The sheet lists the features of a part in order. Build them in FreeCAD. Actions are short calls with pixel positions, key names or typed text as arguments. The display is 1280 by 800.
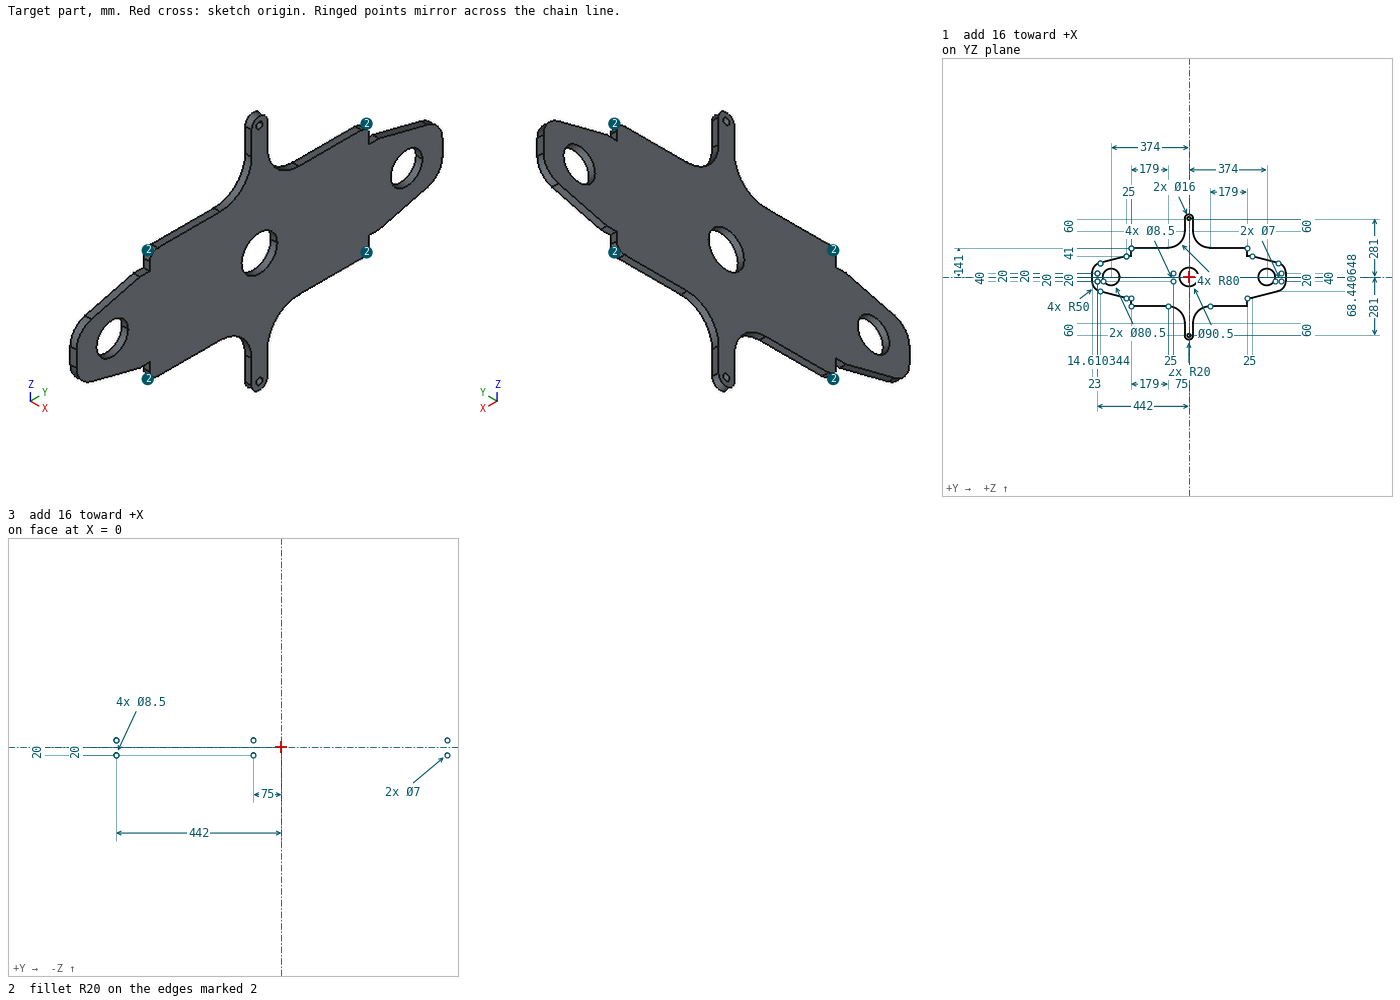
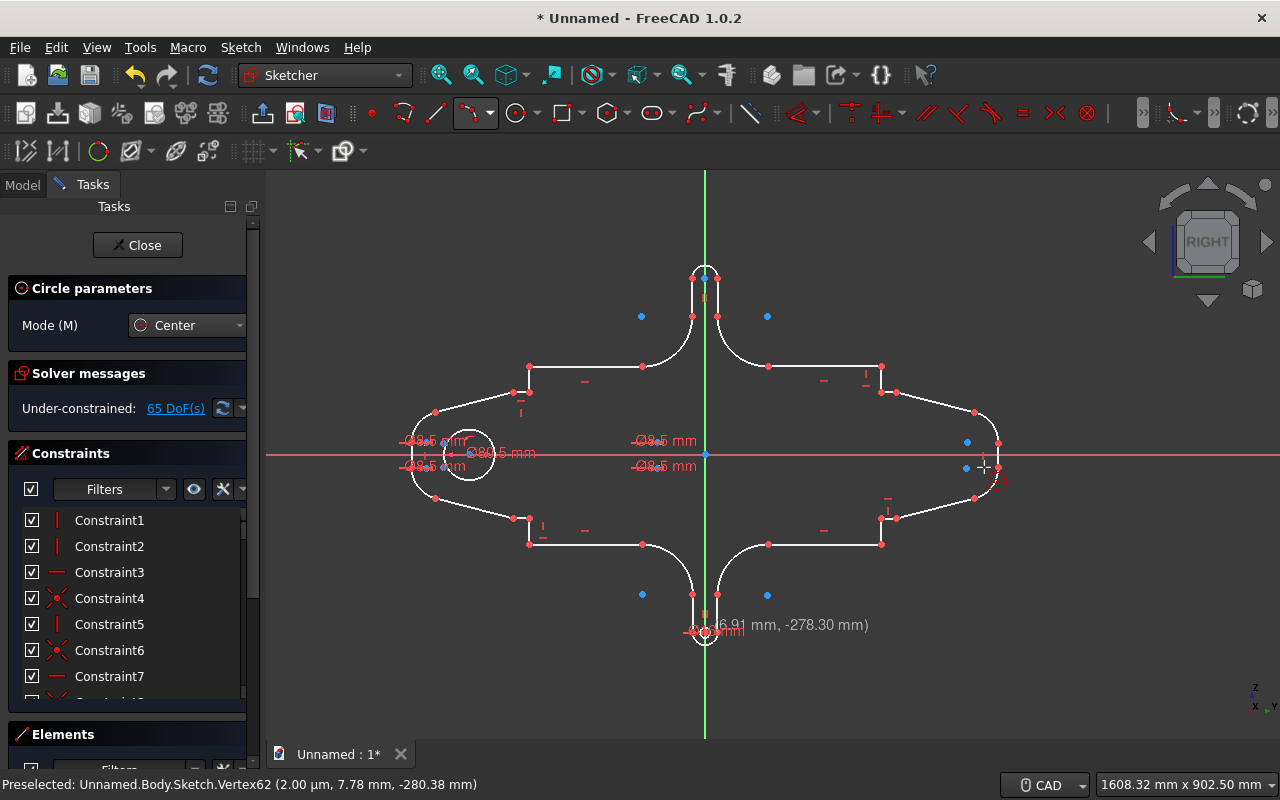
scroll(984, 467, up, 2)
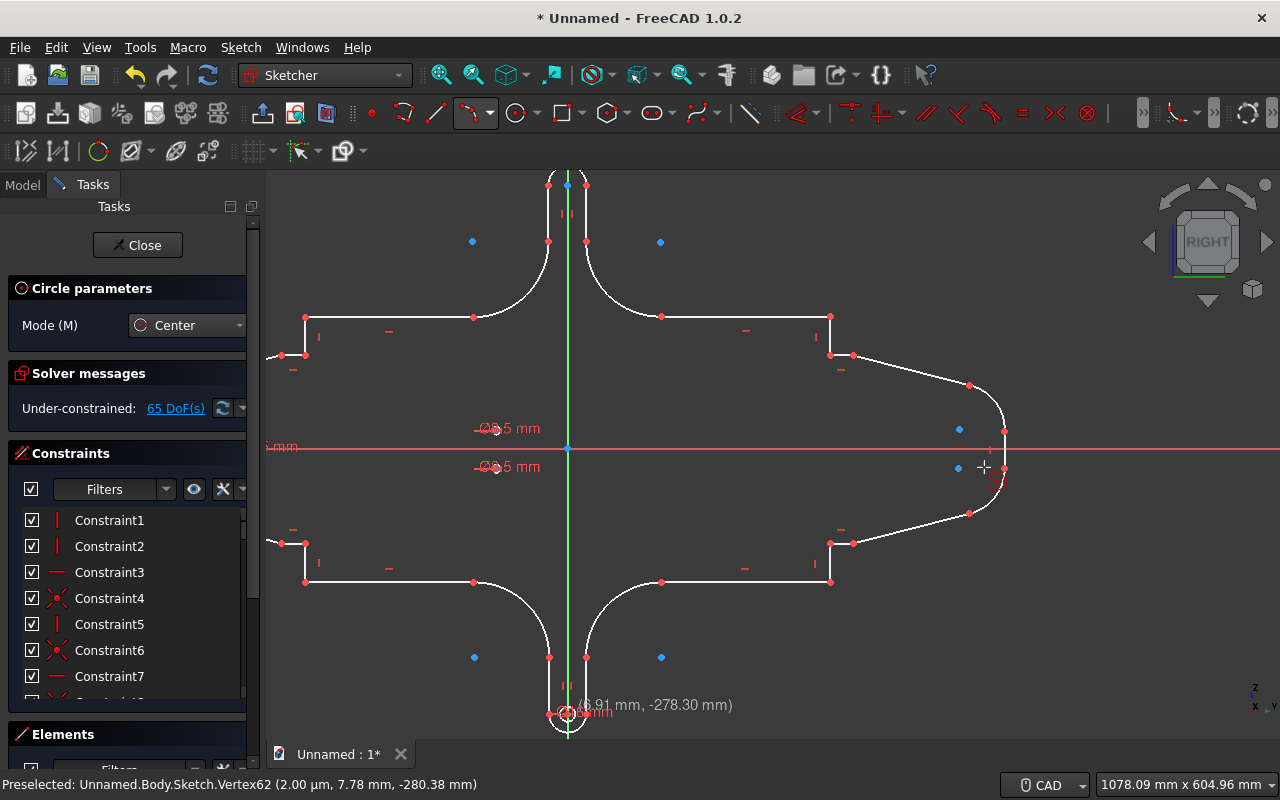
click(983, 467)
move(986, 465)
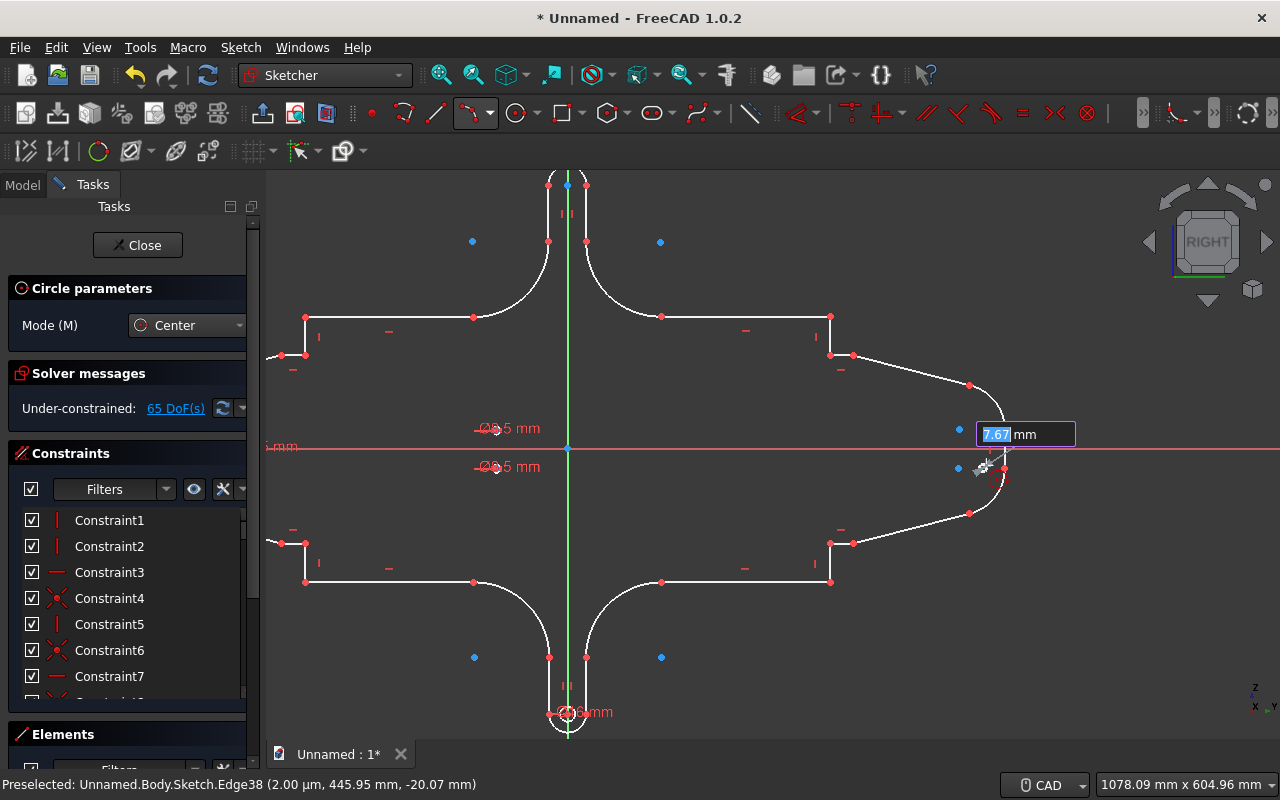
text(7)
key(Return)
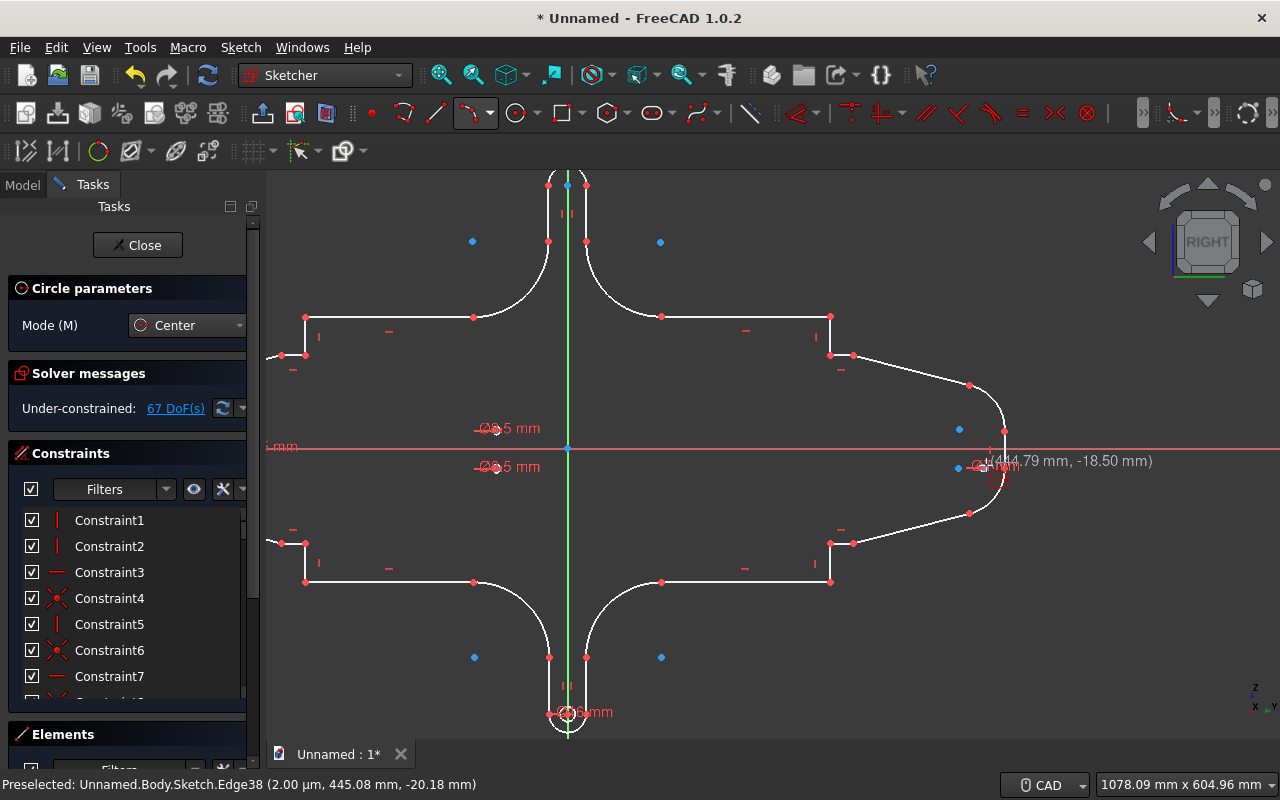
click(568, 449)
move(598, 419)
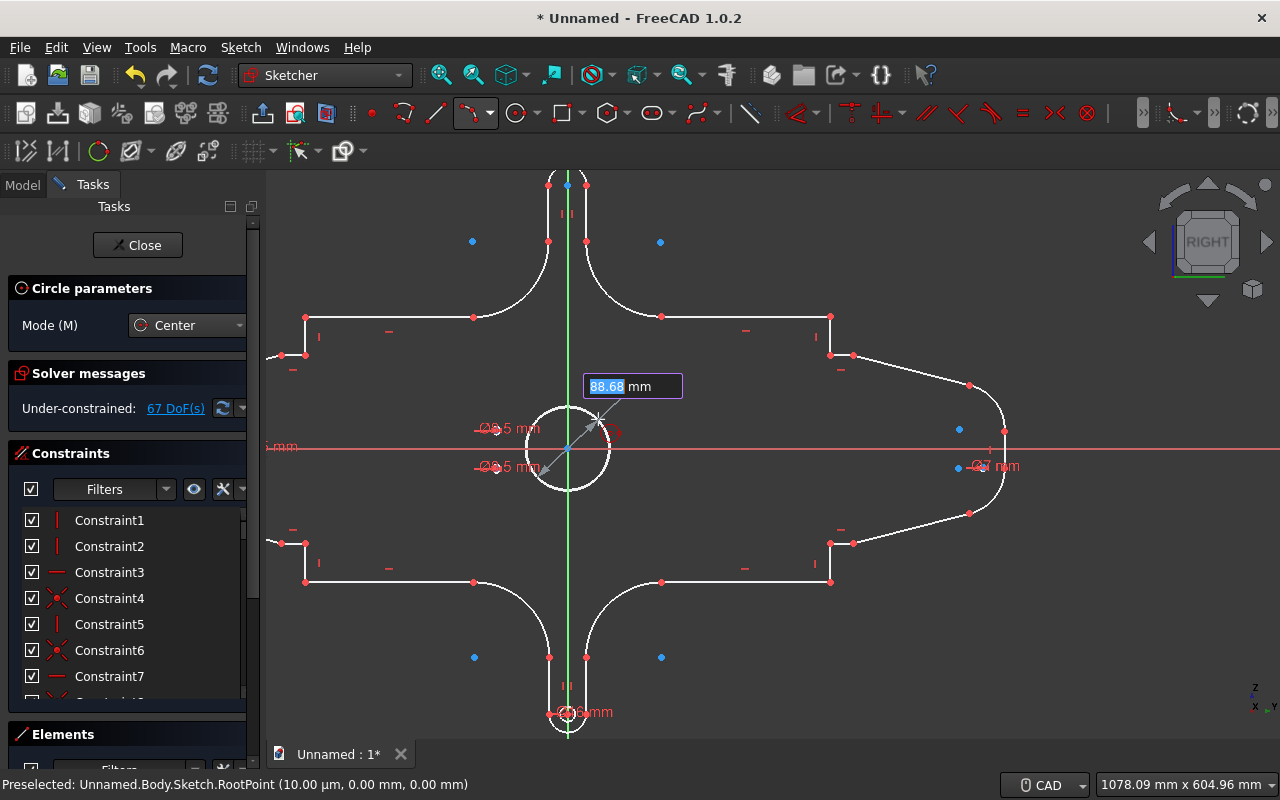
text(90.5)
key(Return)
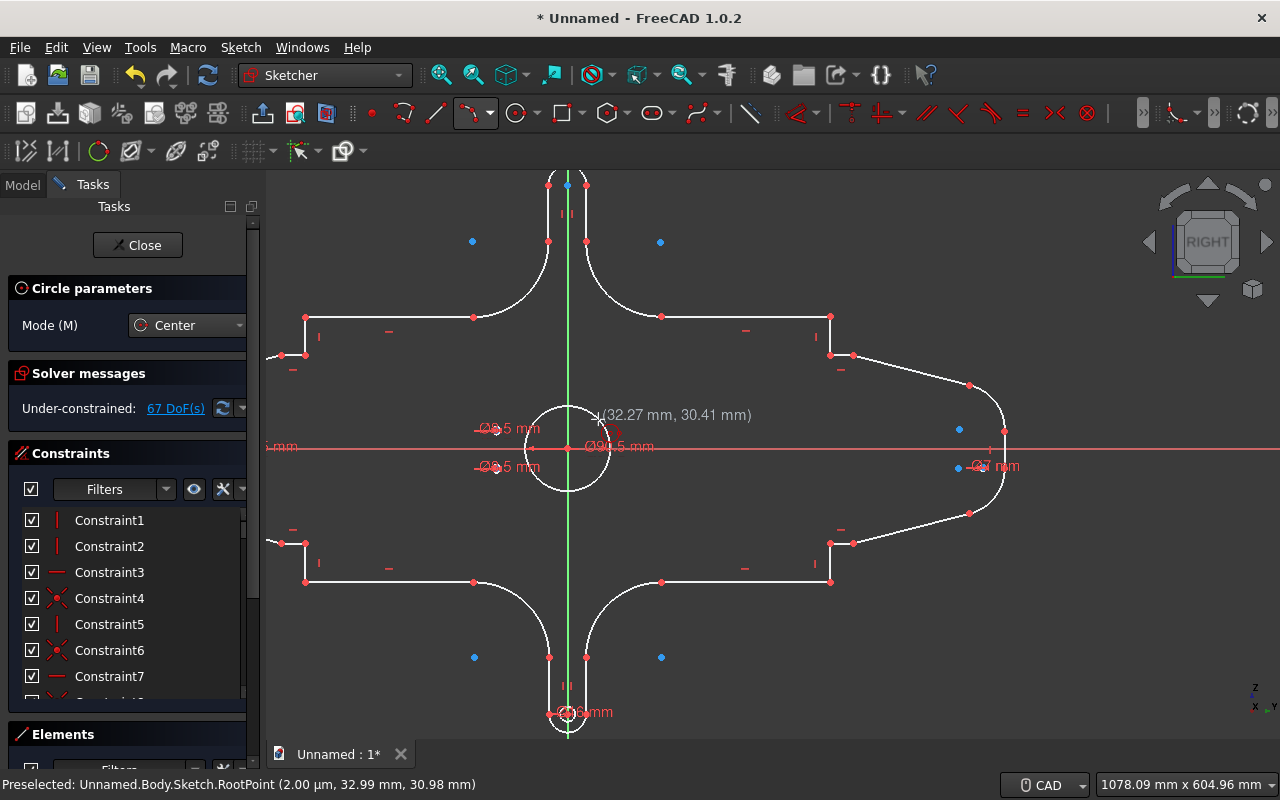
scroll(983, 466, down, 2)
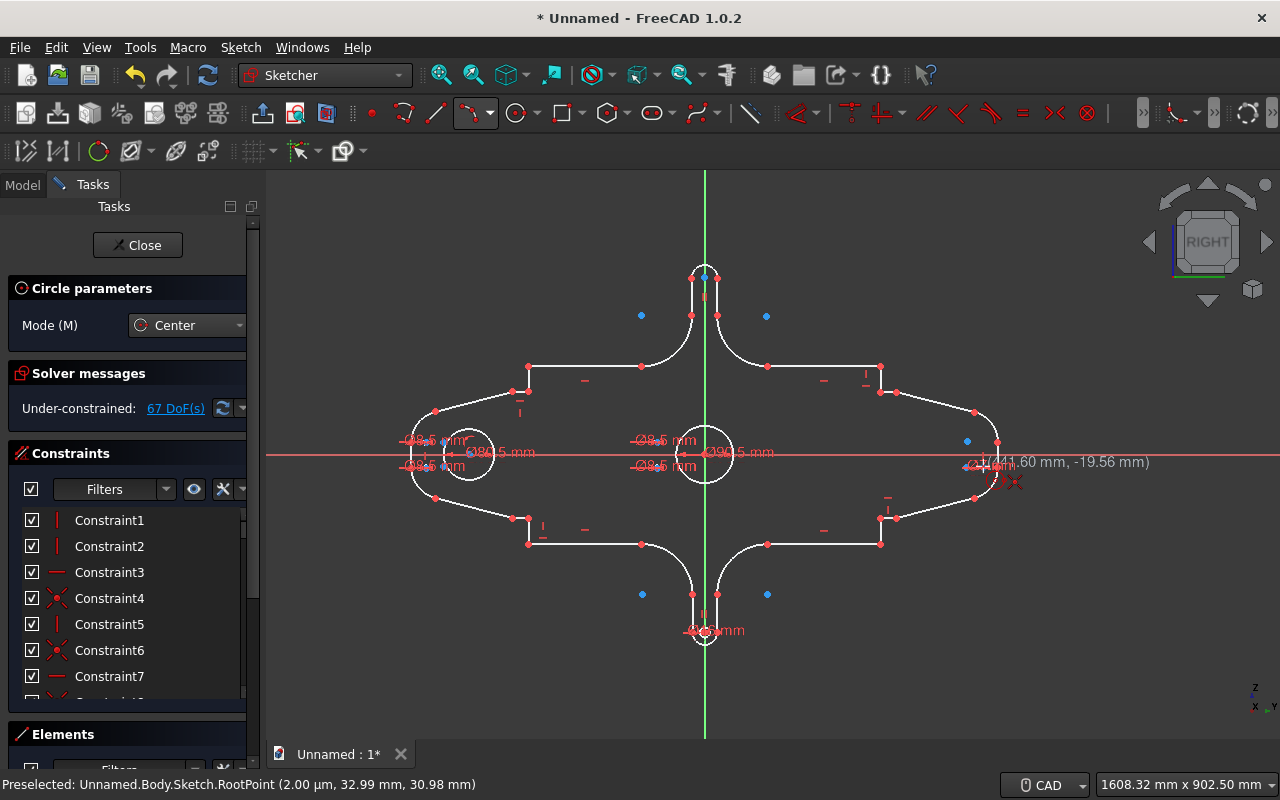
scroll(705, 277, up, 8)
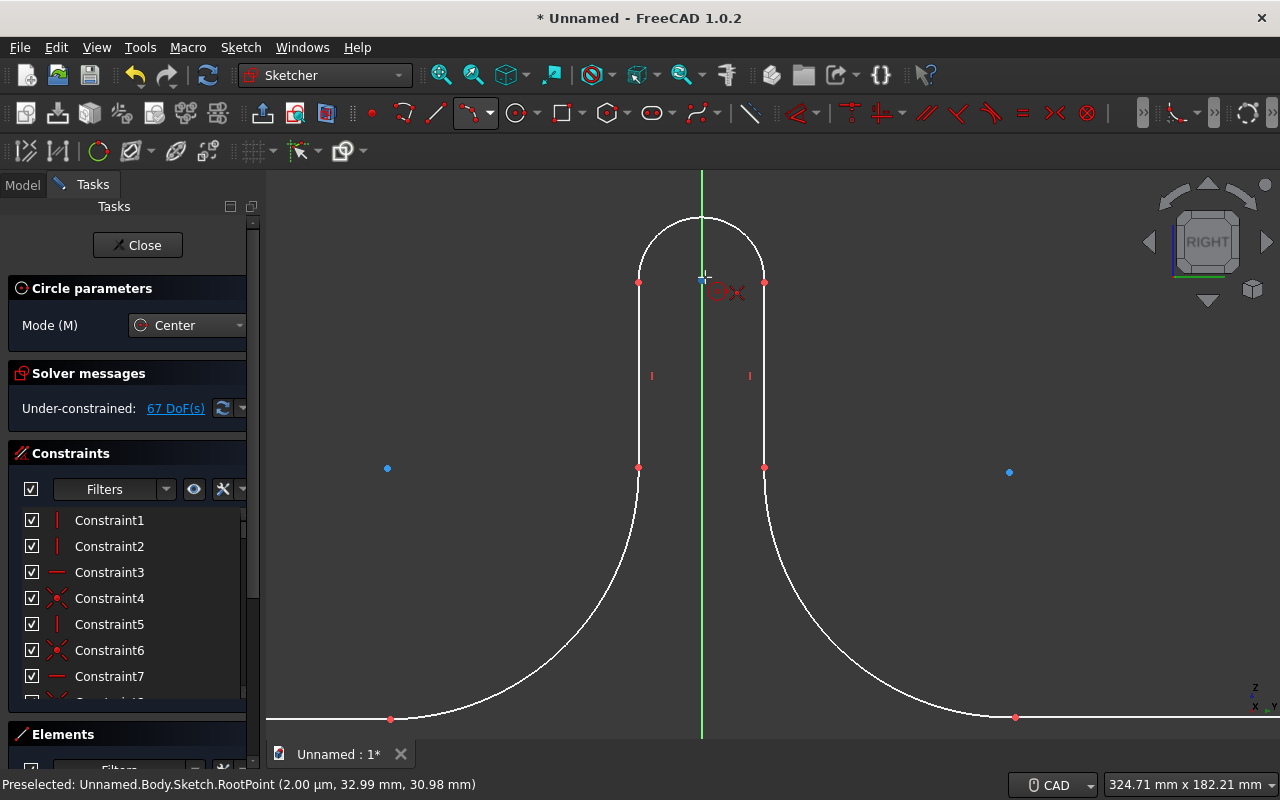
scroll(705, 277, down, 8)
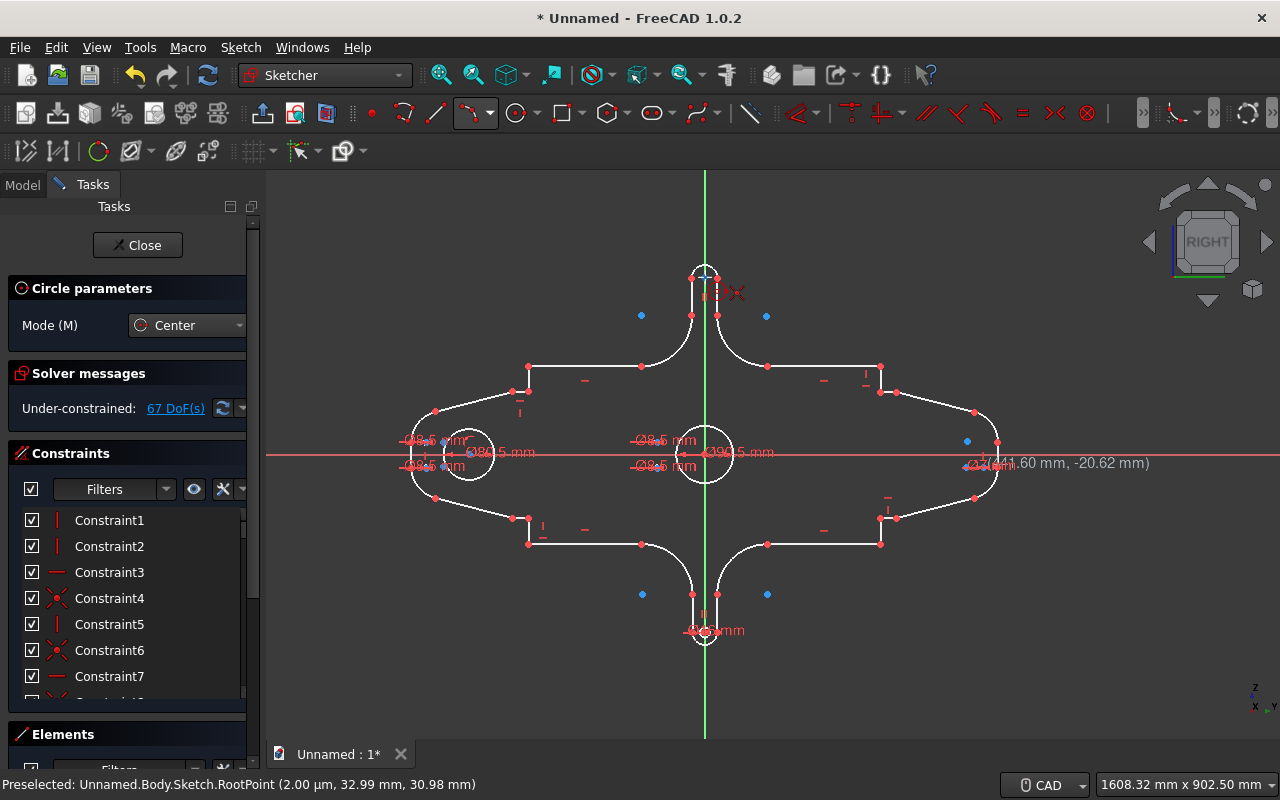
scroll(705, 277, up, 2)